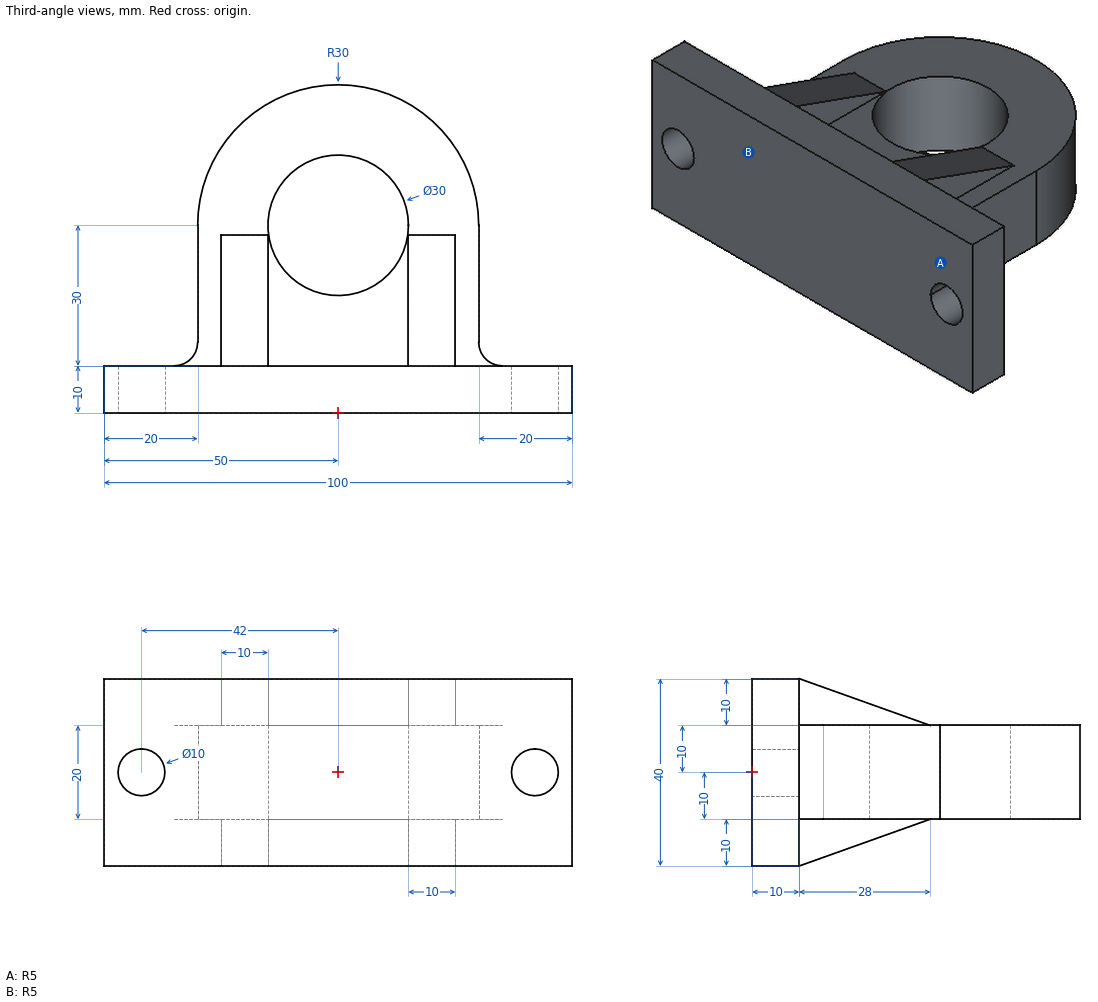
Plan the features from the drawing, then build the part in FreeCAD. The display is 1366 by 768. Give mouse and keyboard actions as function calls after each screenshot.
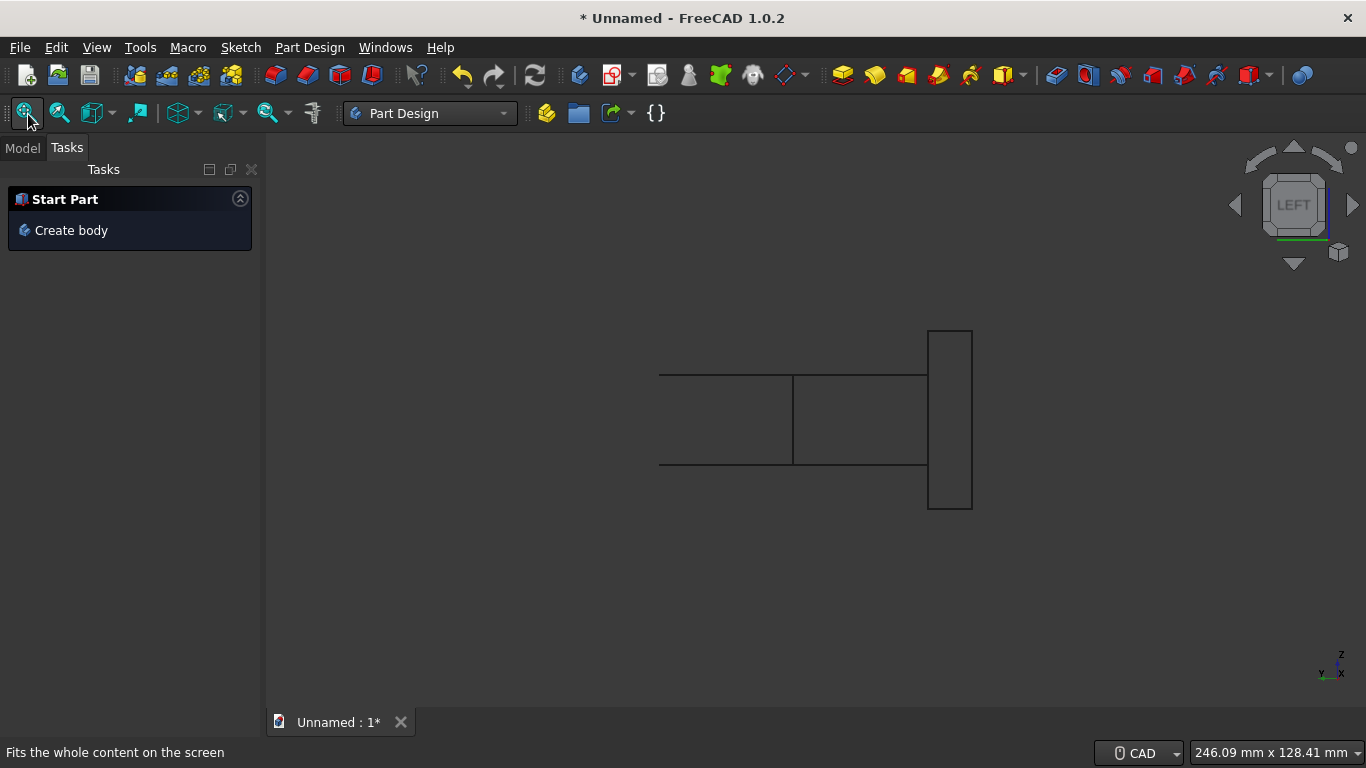
key(0)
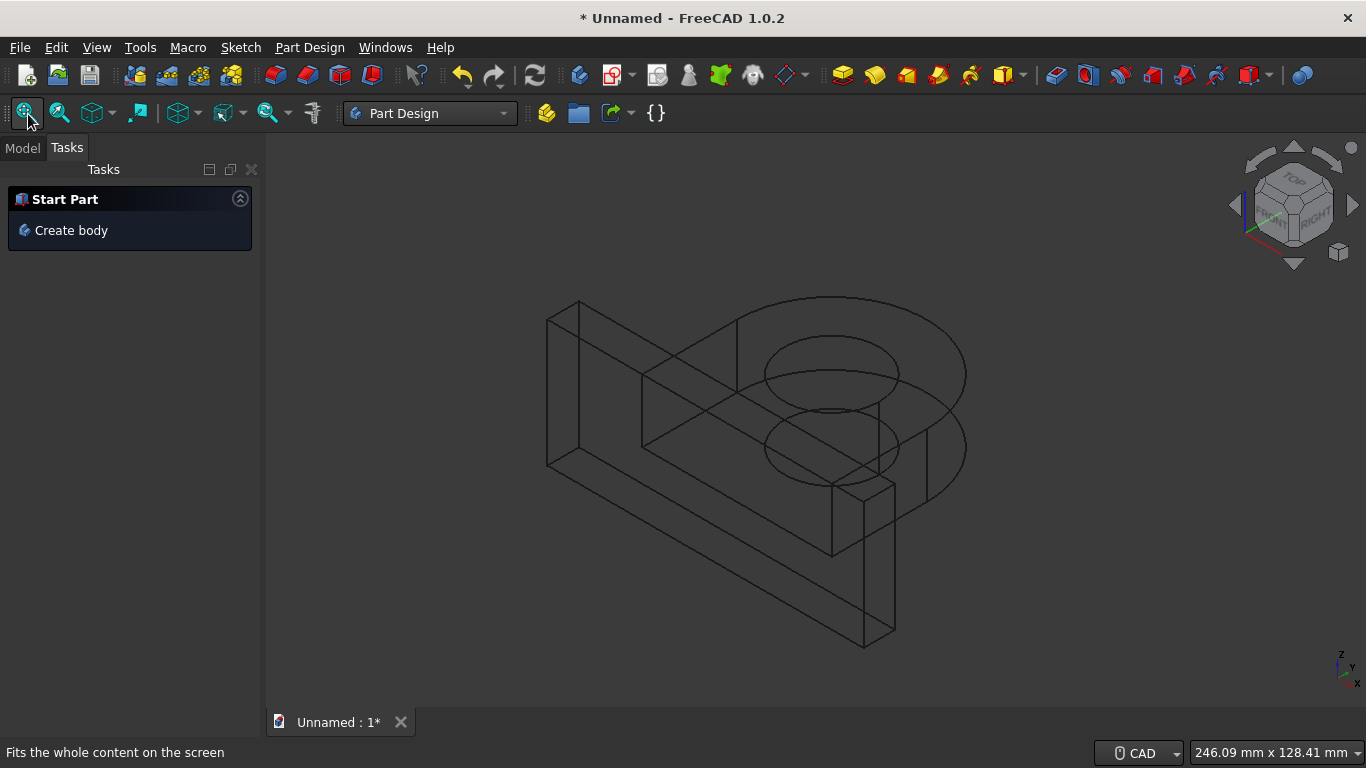
click(832, 519)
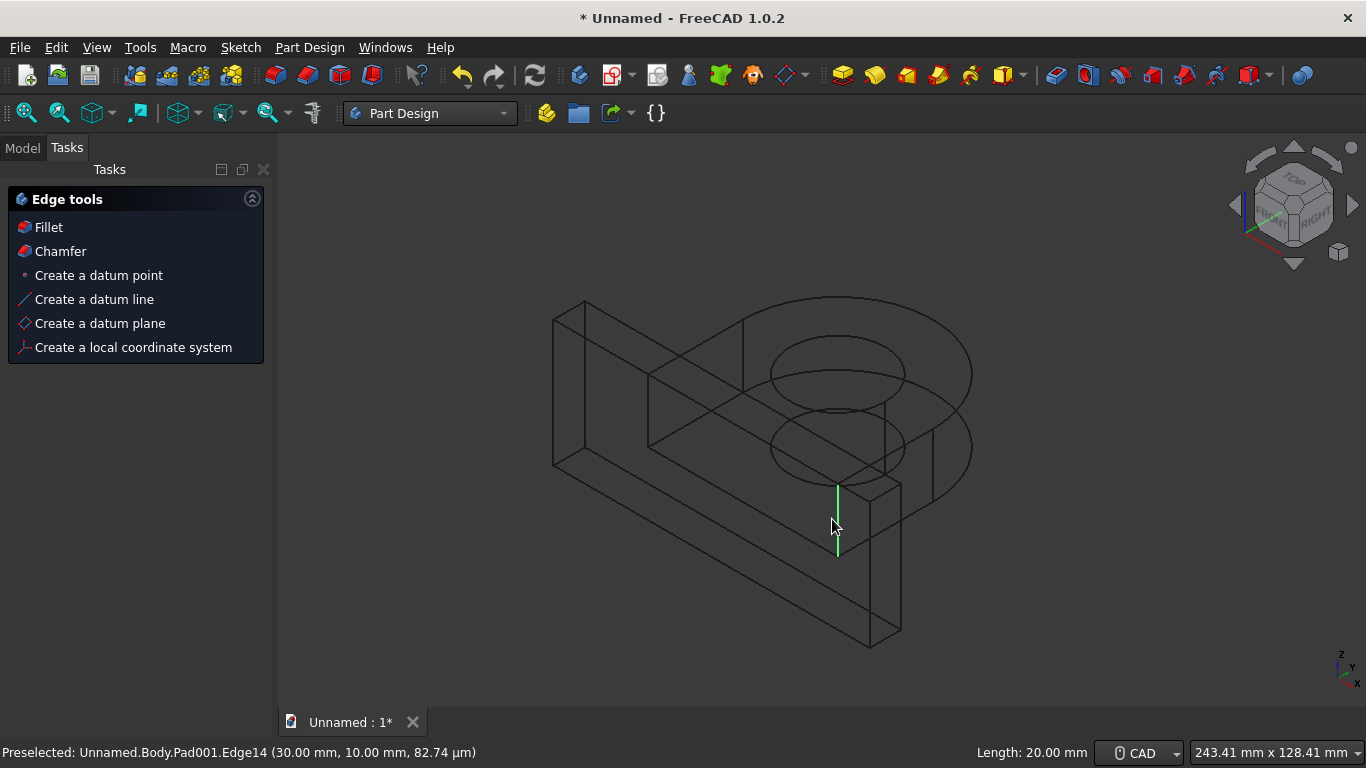
key(v)
key(1)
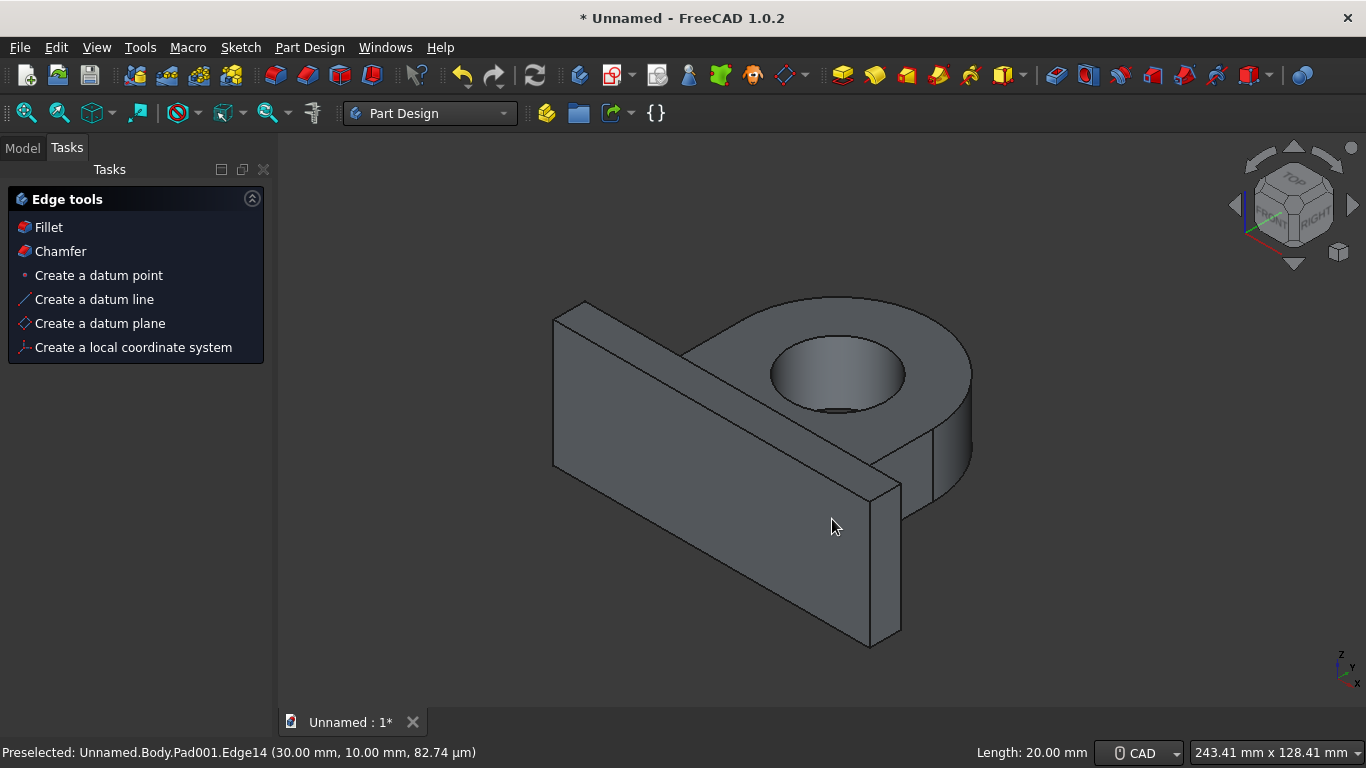
click(276, 76)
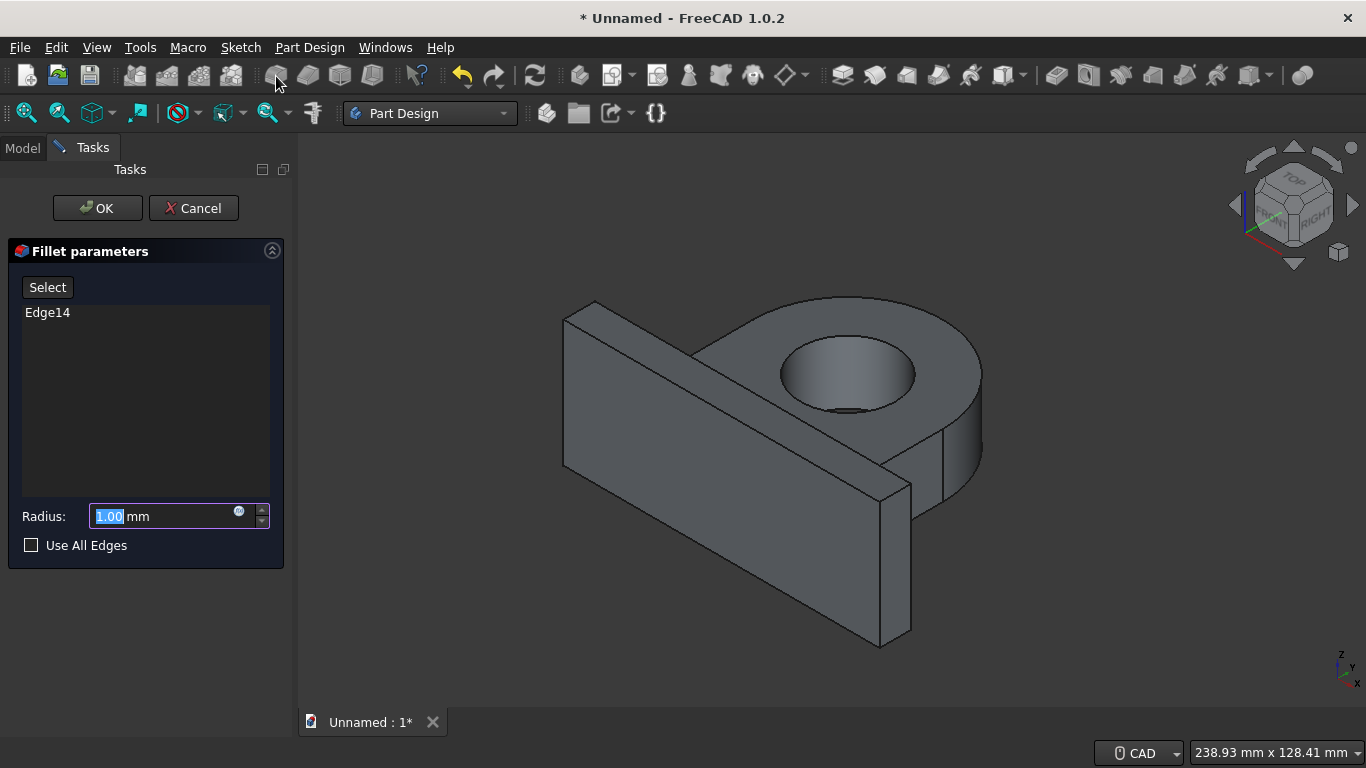
text(5)
key(Tab)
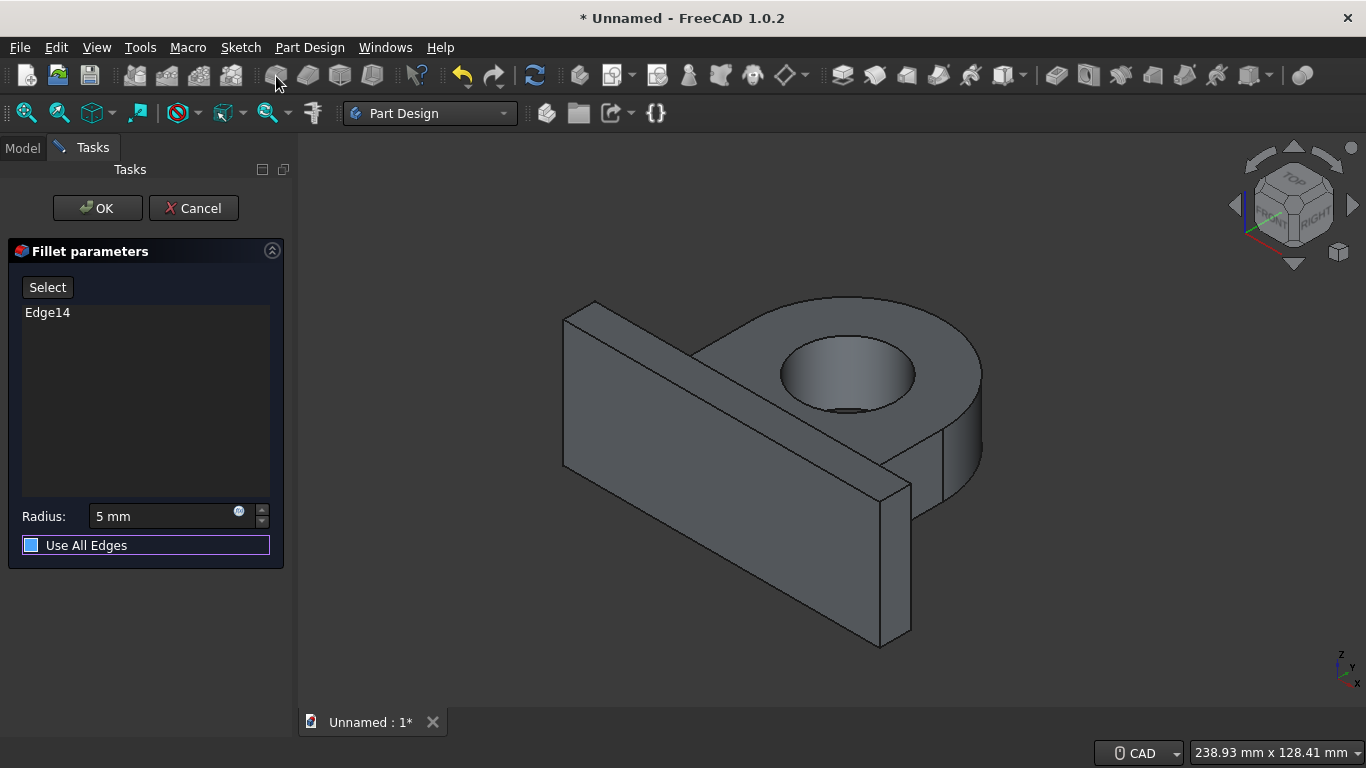
click(98, 208)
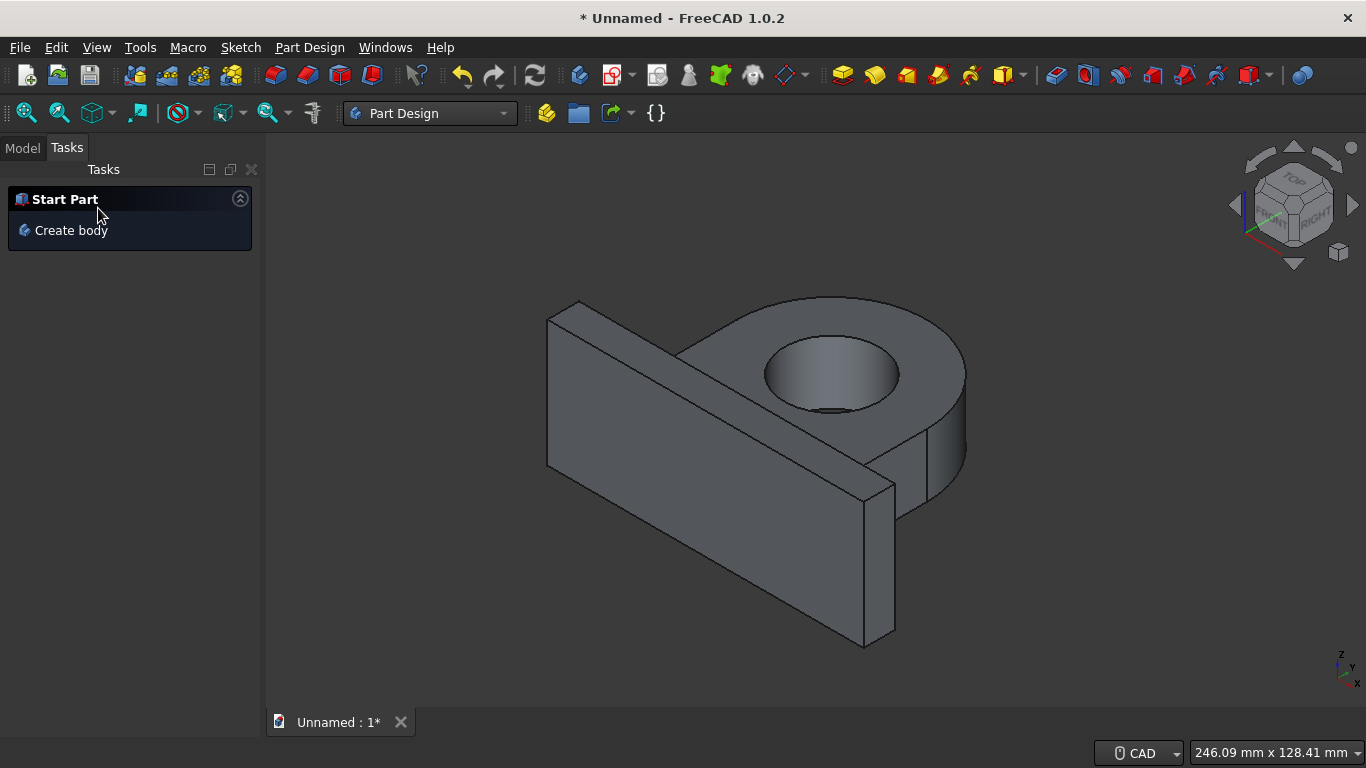
key(2)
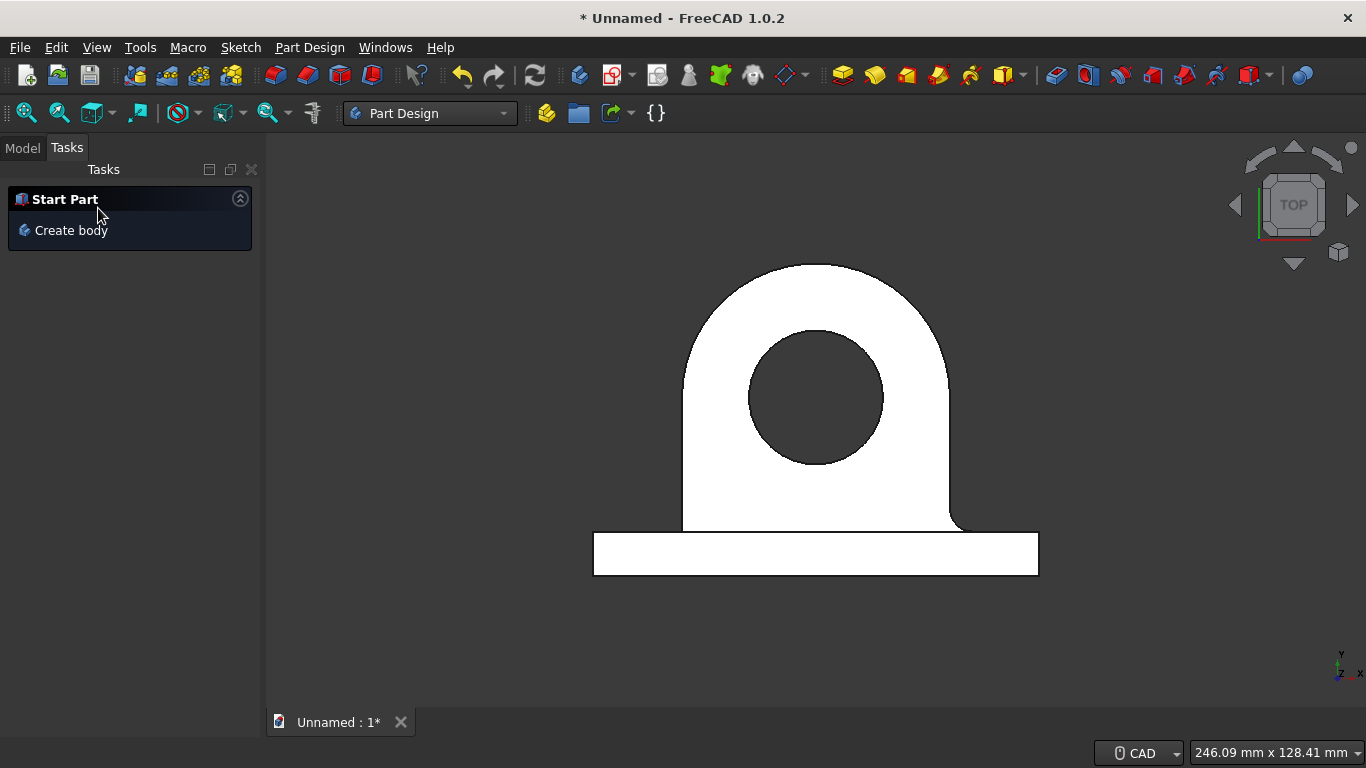
key(0)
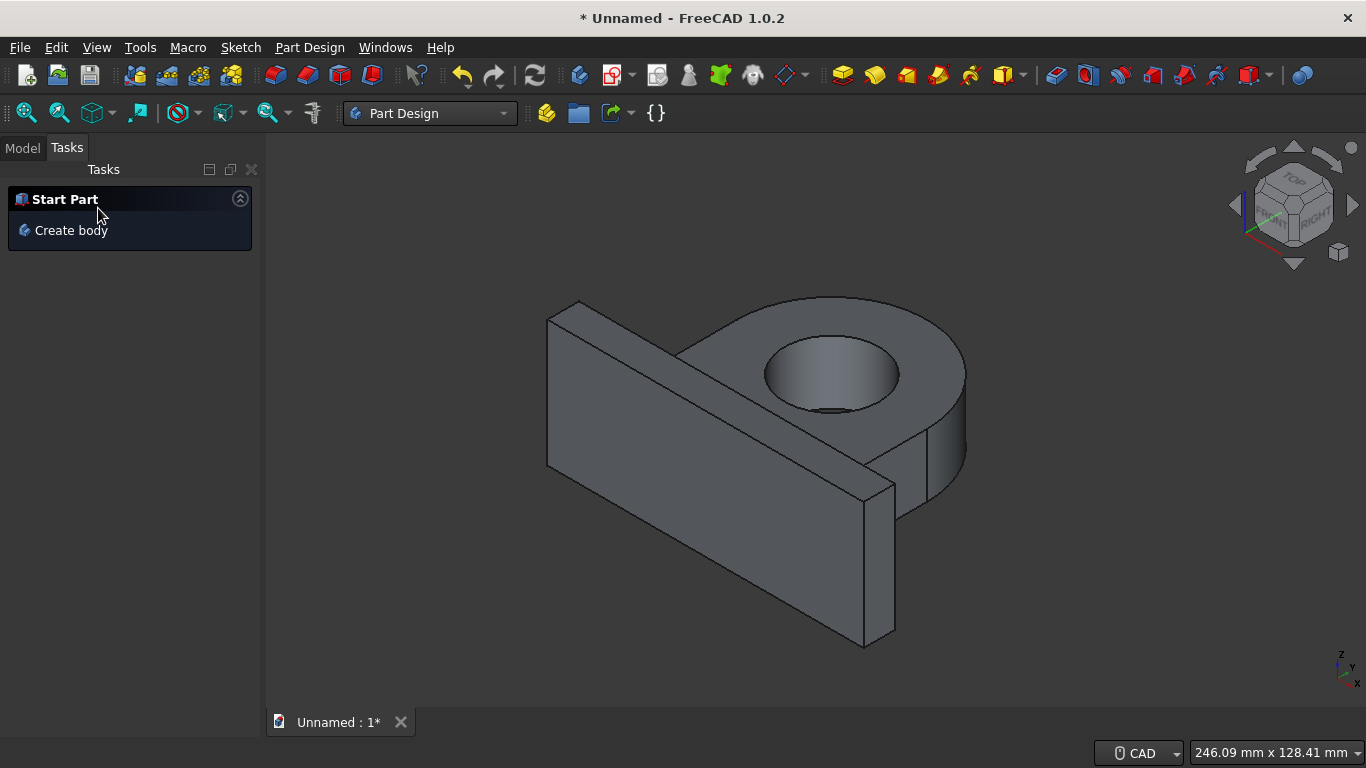
key(1)